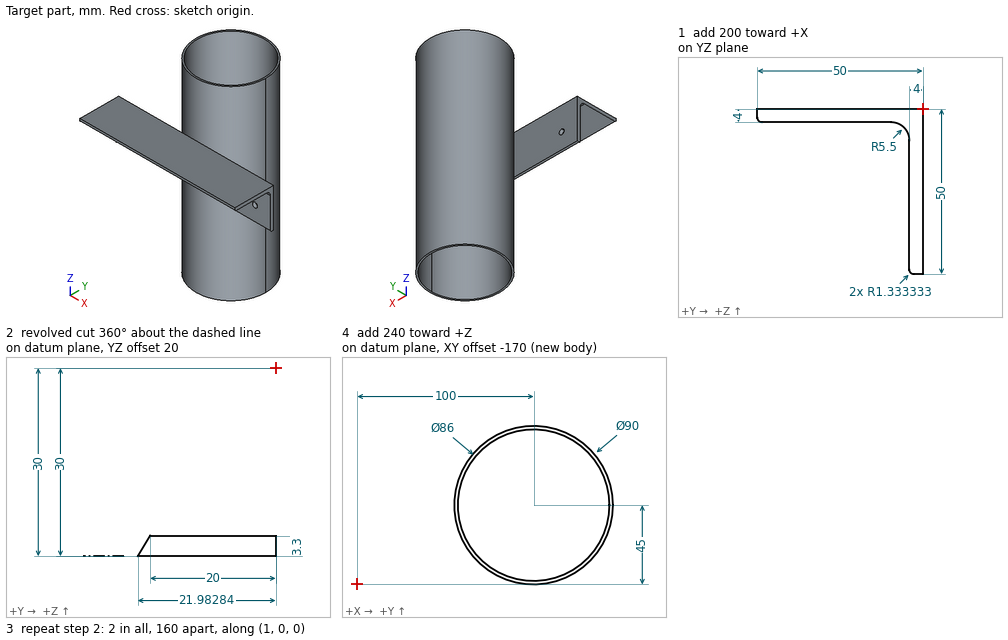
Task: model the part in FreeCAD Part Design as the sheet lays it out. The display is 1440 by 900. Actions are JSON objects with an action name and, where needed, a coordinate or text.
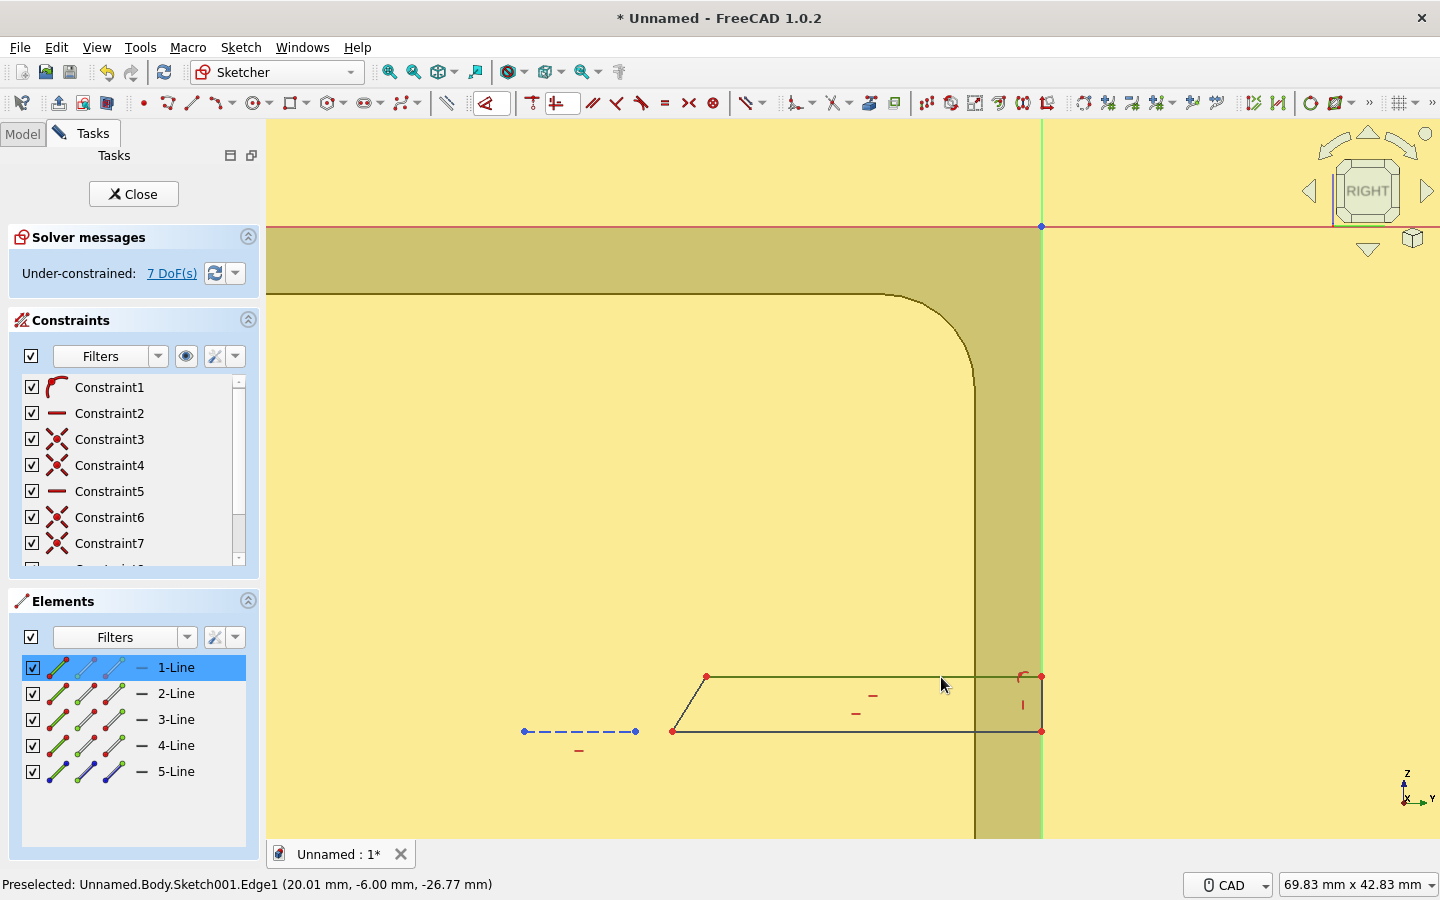
{"action": "key", "text": "l"}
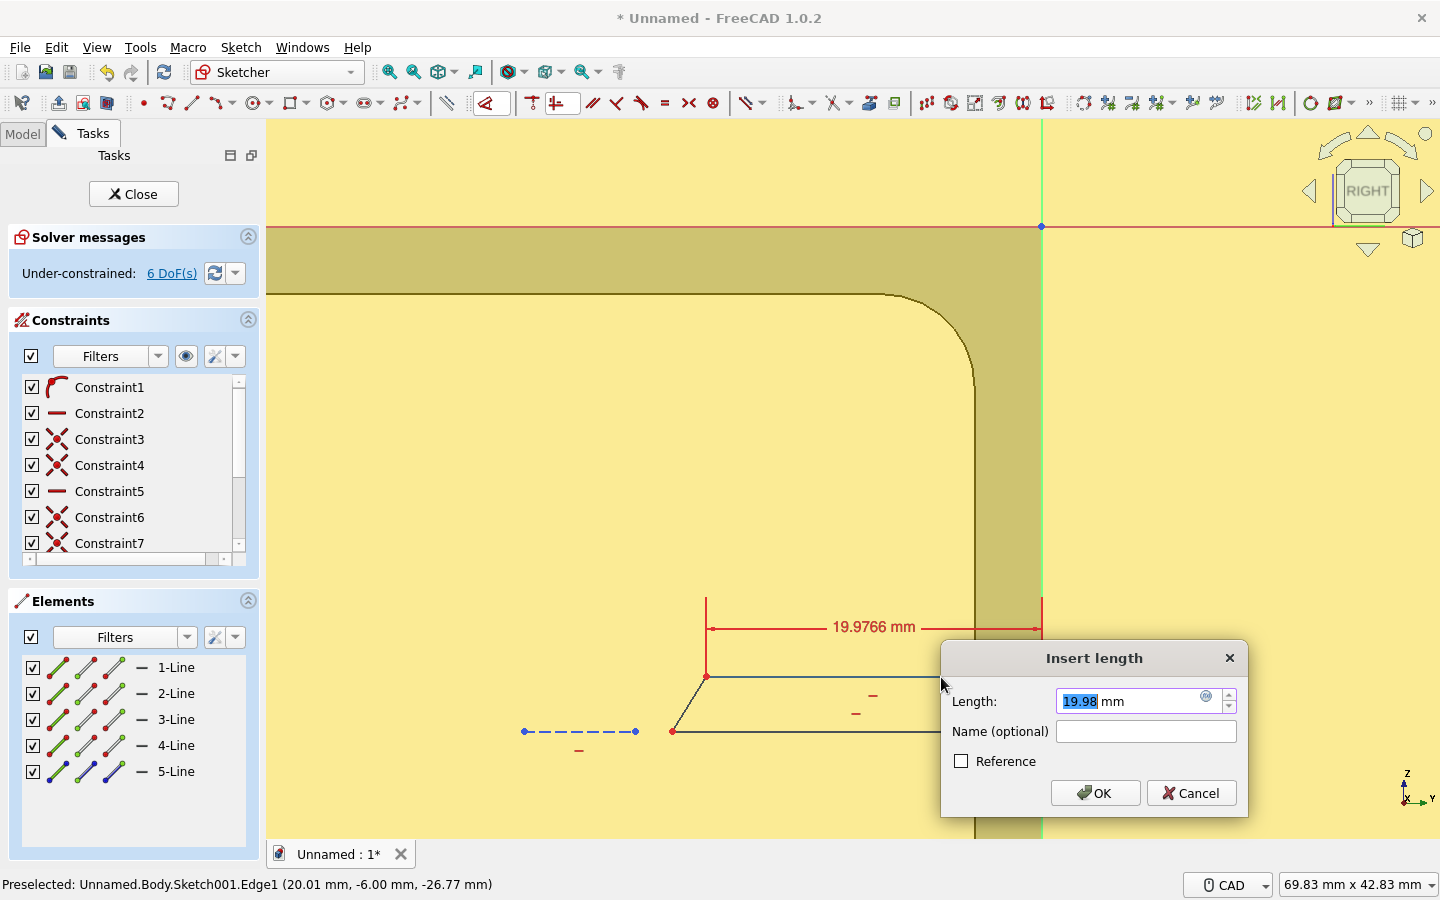
{"action": "type", "text": "20"}
{"action": "key", "text": "Return"}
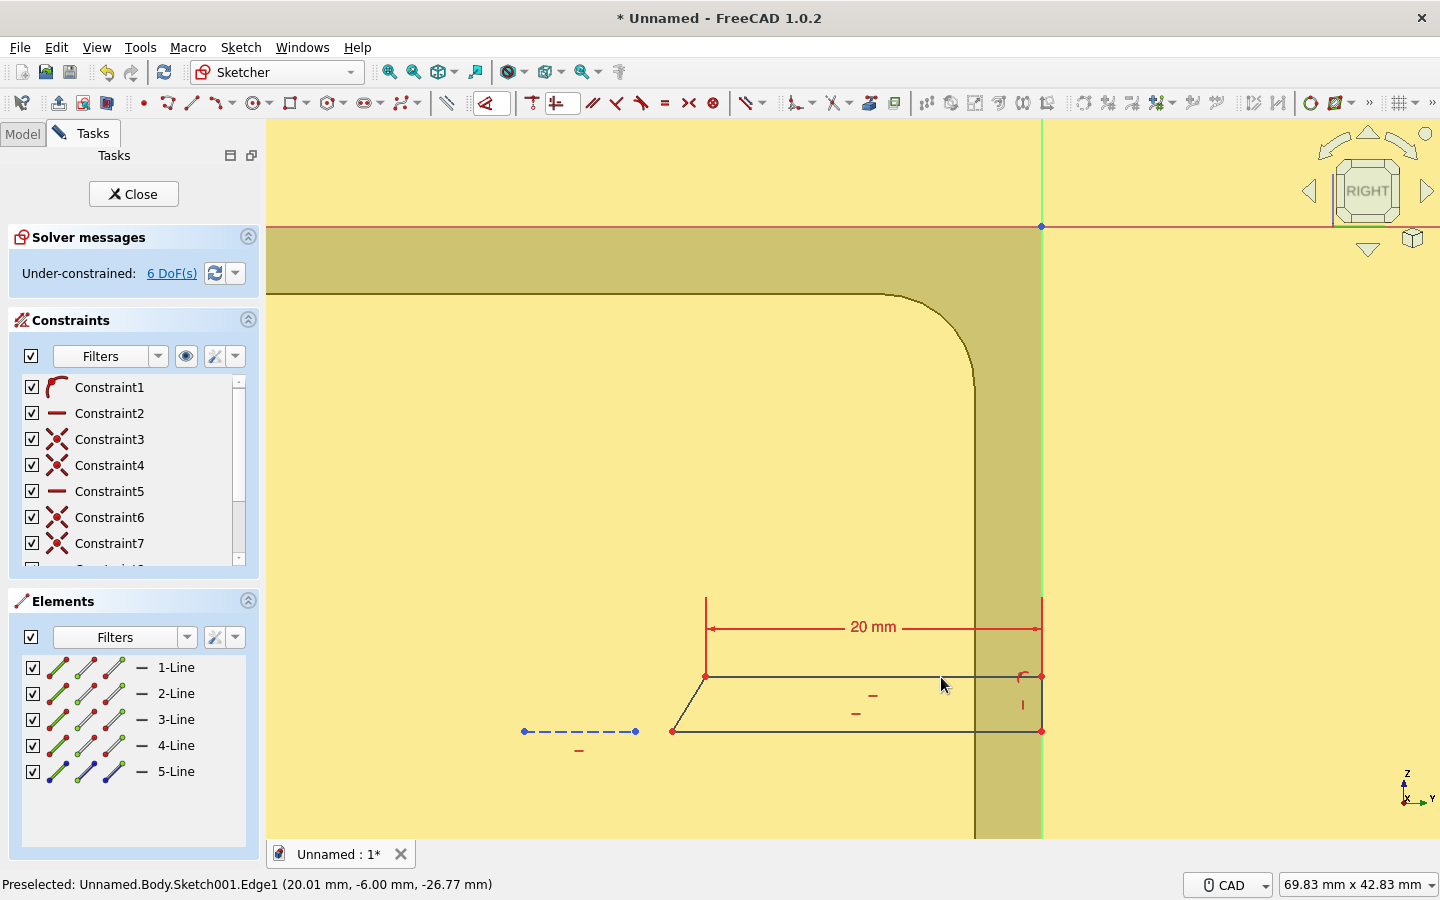
{"action": "left_click", "coordinate": [1042, 716]}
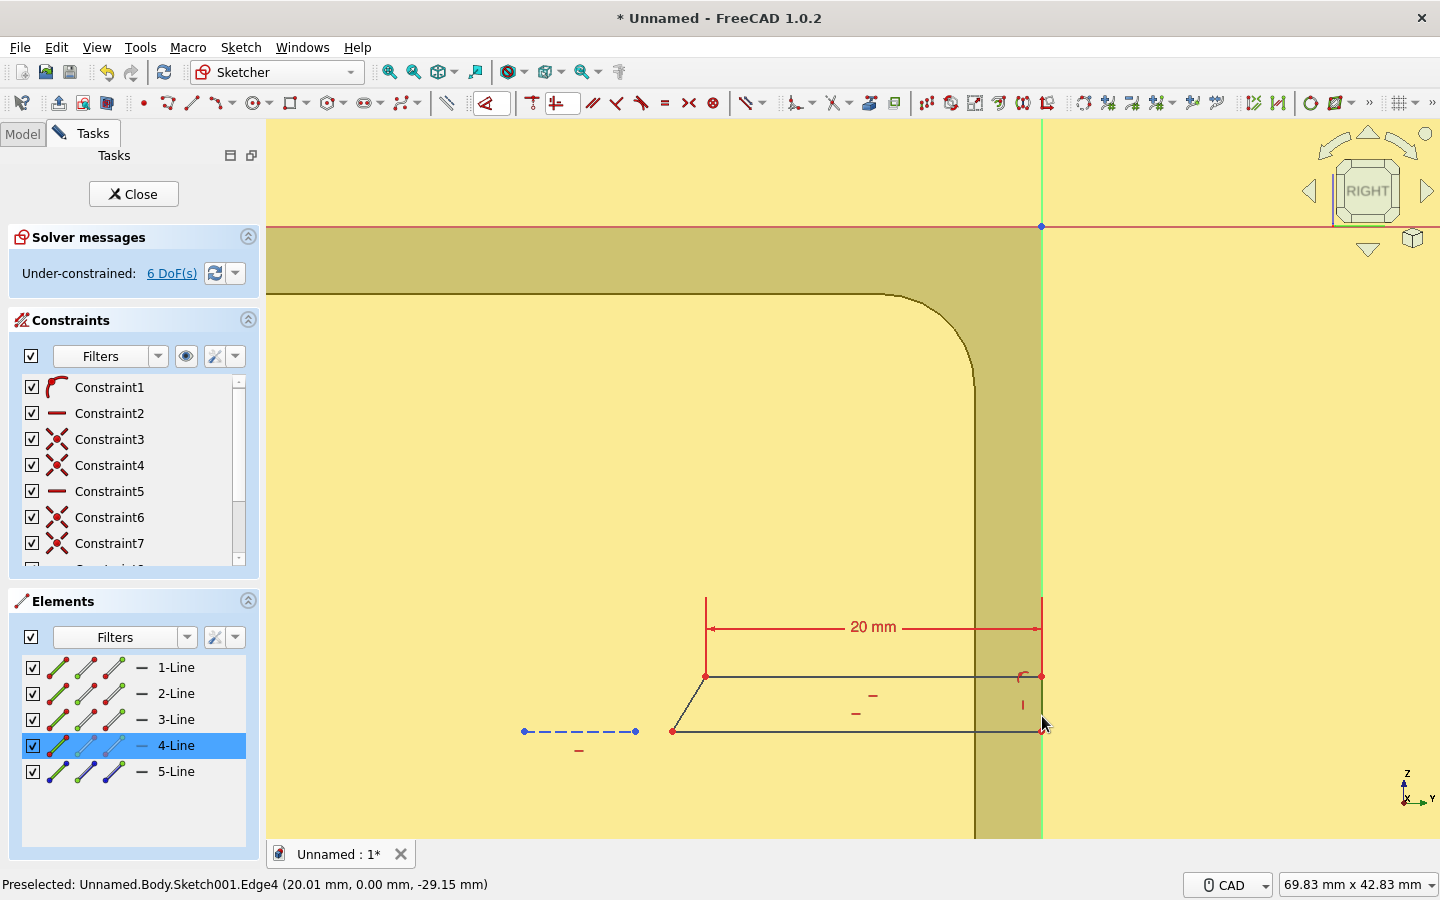
{"action": "left_click", "coordinate": [504, 104]}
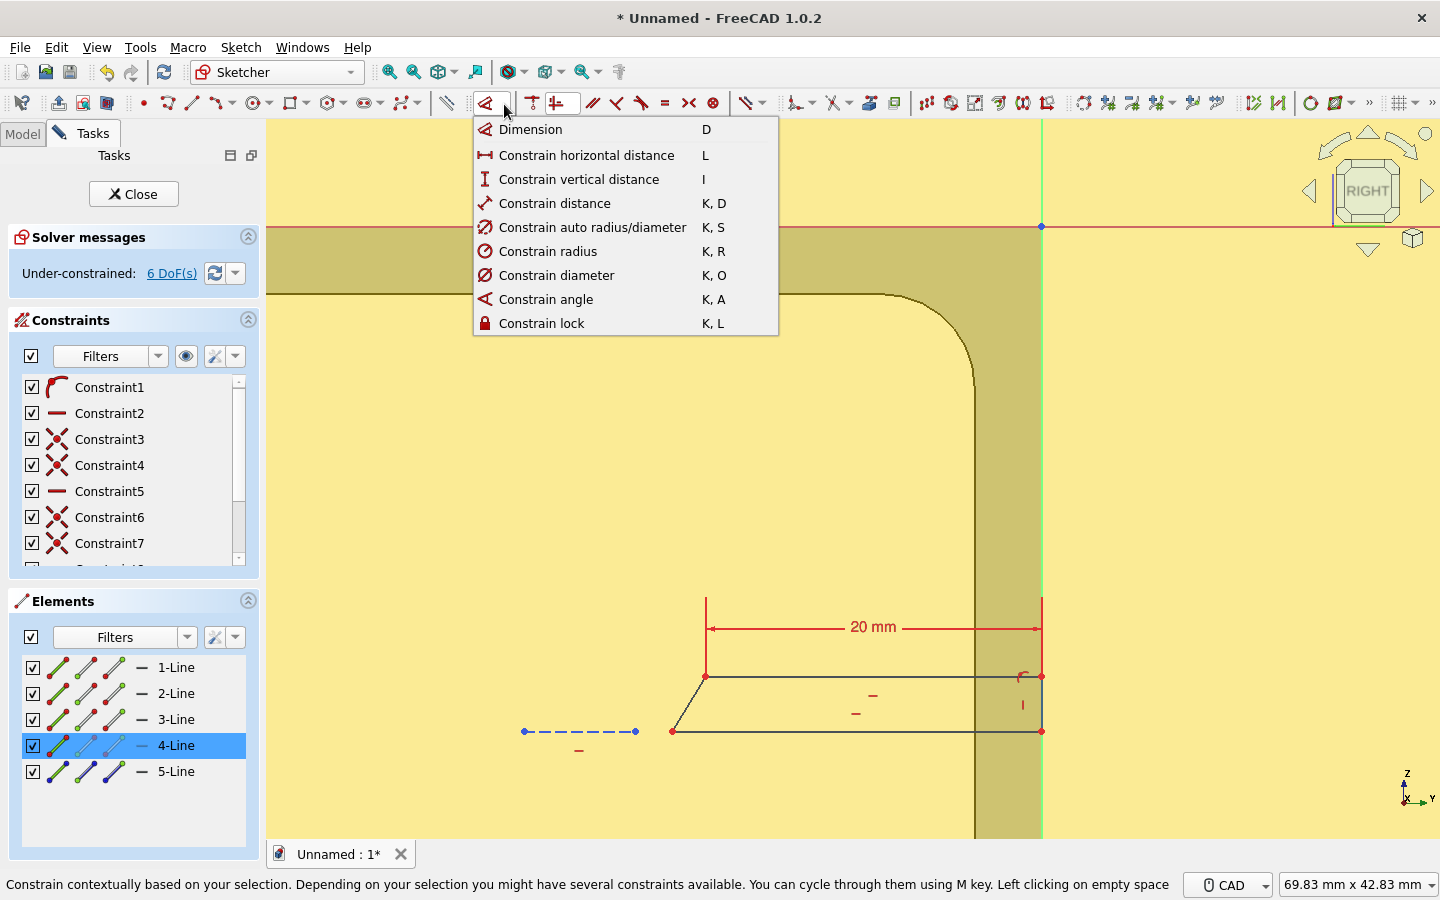
{"action": "left_click", "coordinate": [626, 179]}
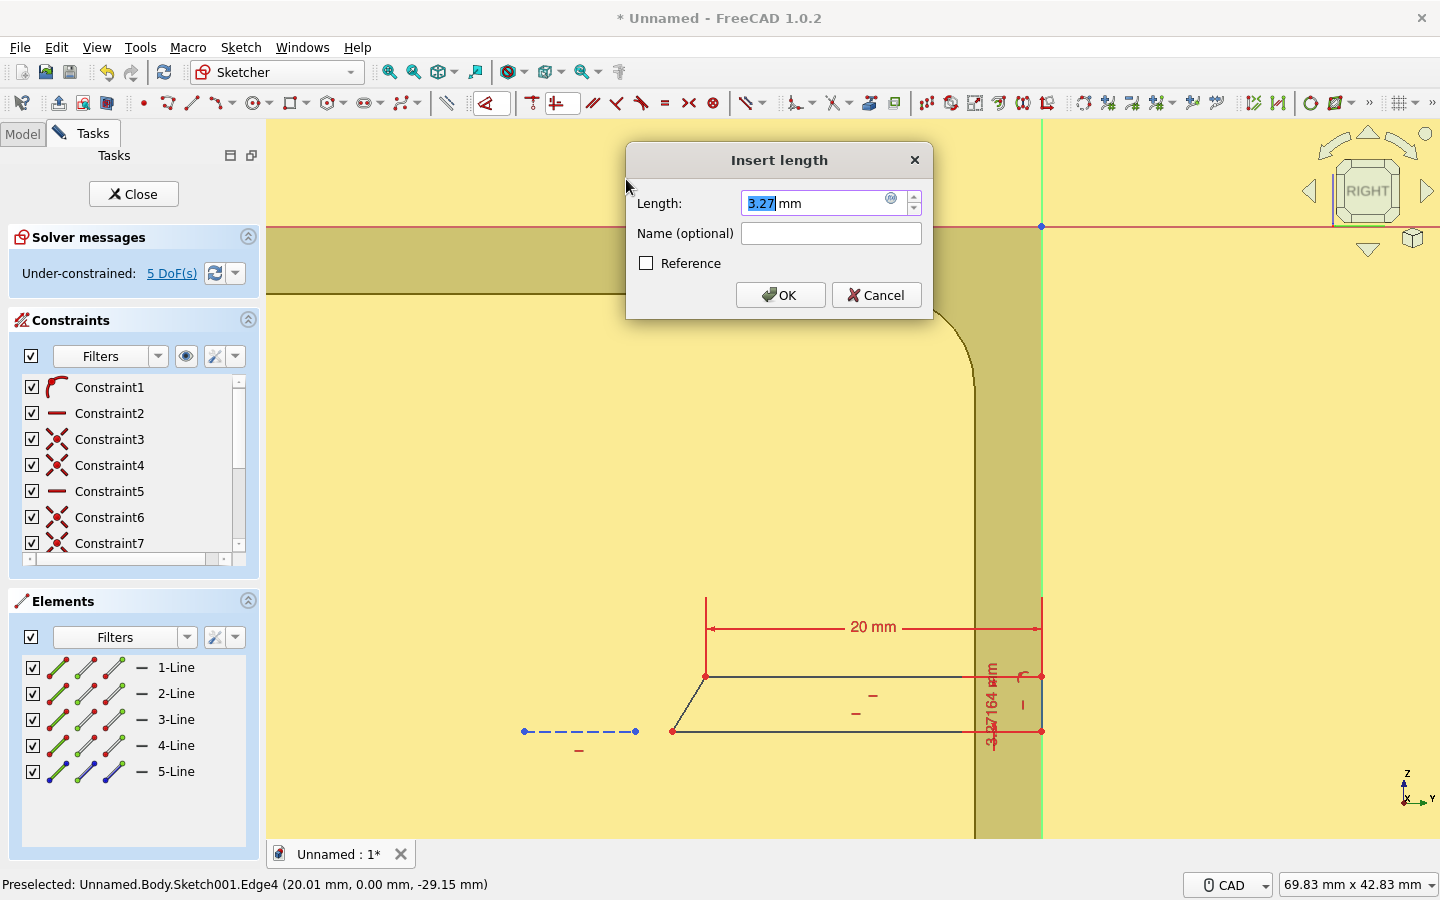
{"action": "type", "text": "3.3"}
{"action": "key", "text": "Return"}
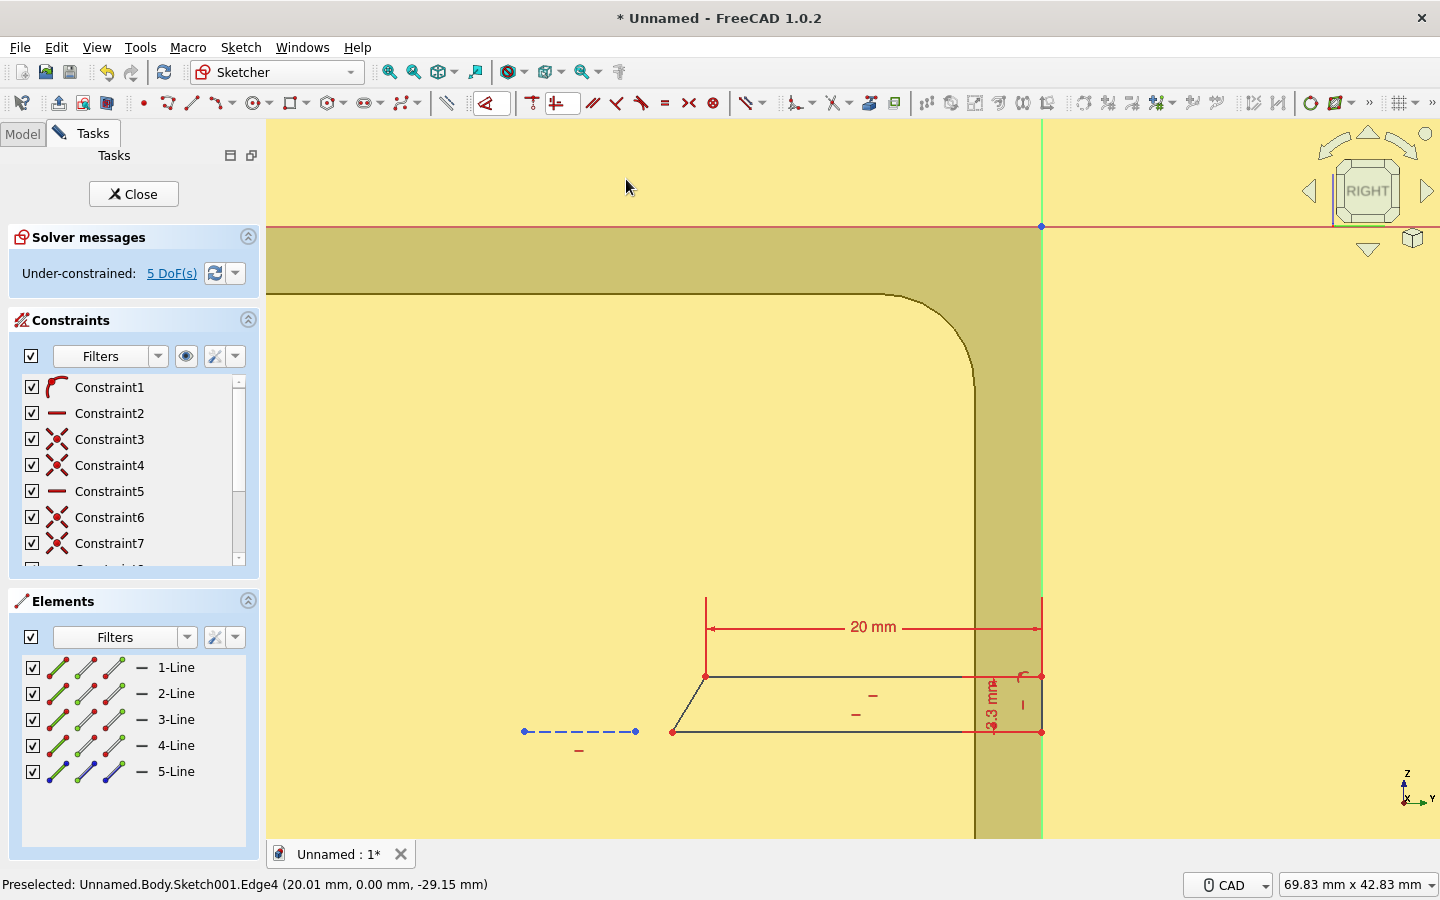
{"action": "left_click", "coordinate": [672, 732]}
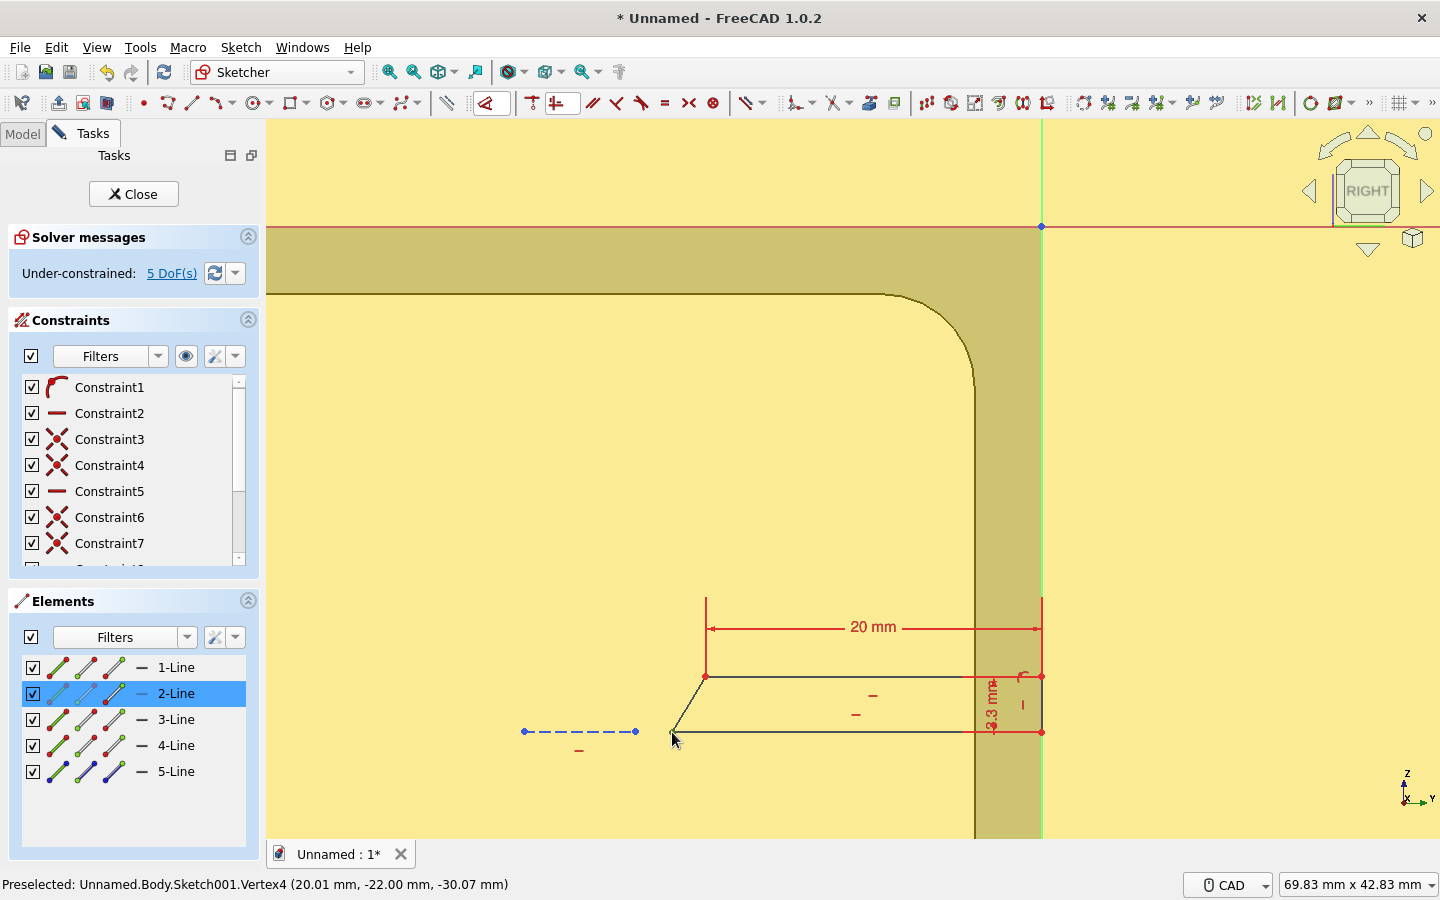
{"action": "left_click", "coordinate": [504, 104]}